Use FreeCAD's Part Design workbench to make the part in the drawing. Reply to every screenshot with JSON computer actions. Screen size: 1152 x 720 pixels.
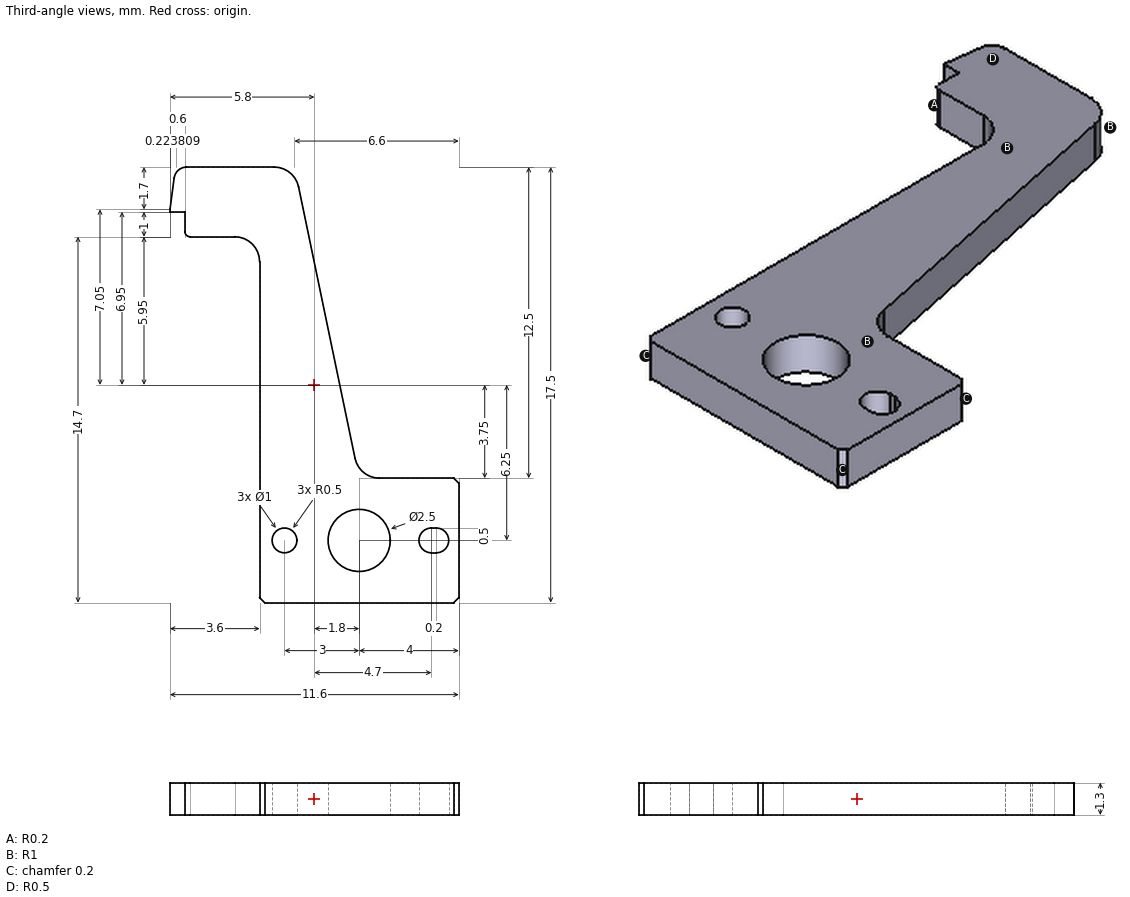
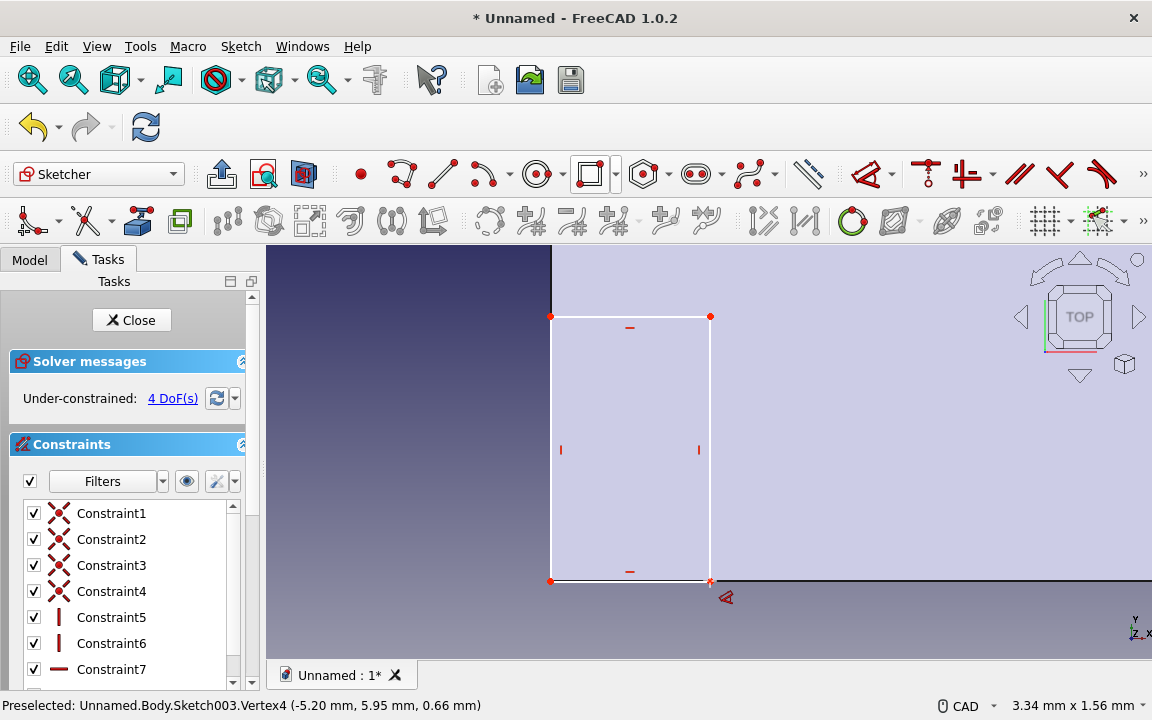
{"action": "left_click", "coordinate": [551, 396]}
{"action": "left_click", "coordinate": [517, 449]}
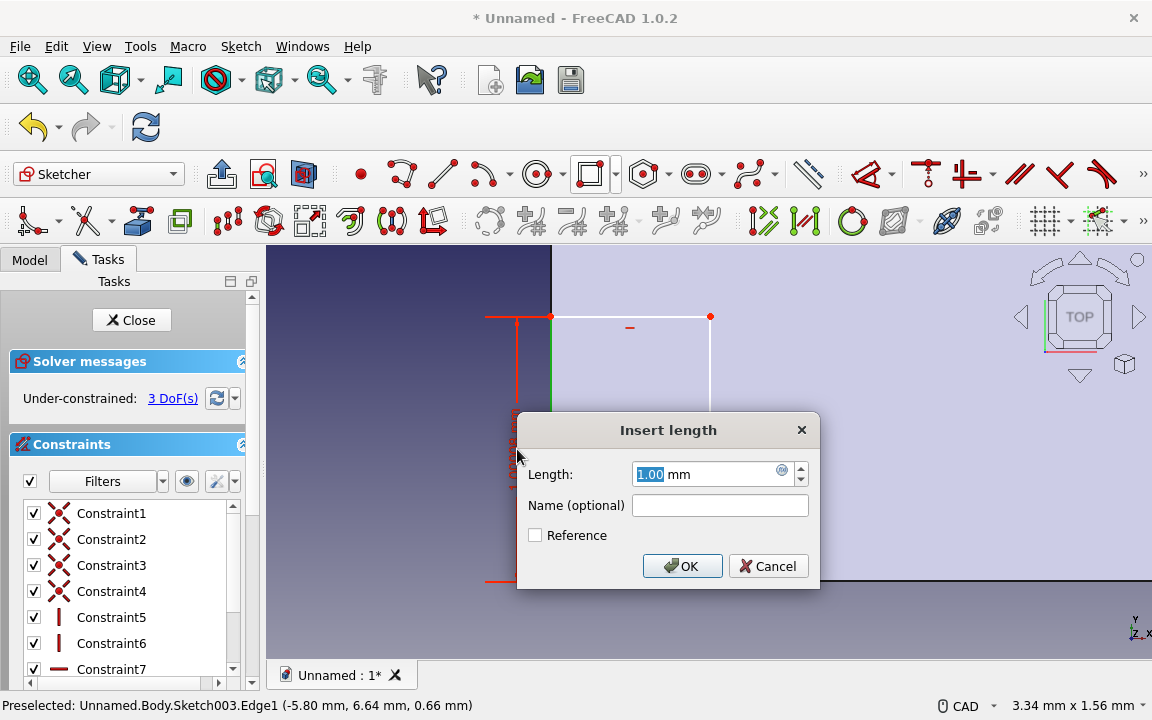
{"action": "type", "text": "1"}
{"action": "key", "text": "Return"}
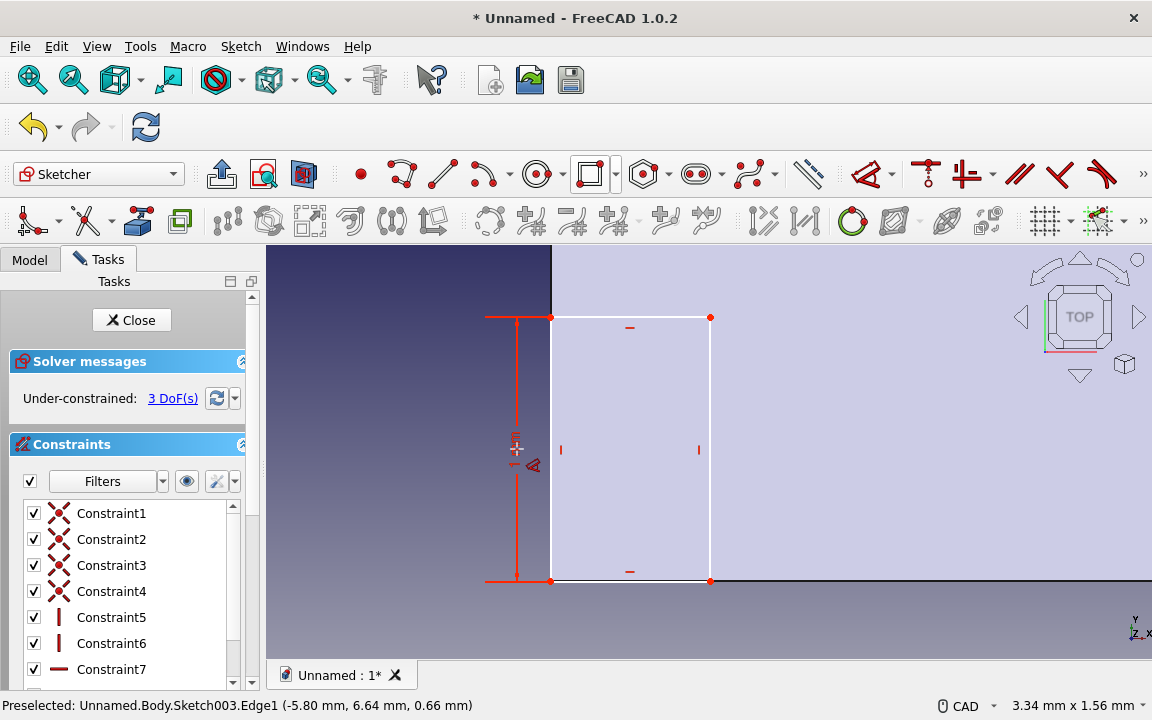
{"action": "left_click", "coordinate": [599, 582]}
{"action": "left_click", "coordinate": [630, 616]}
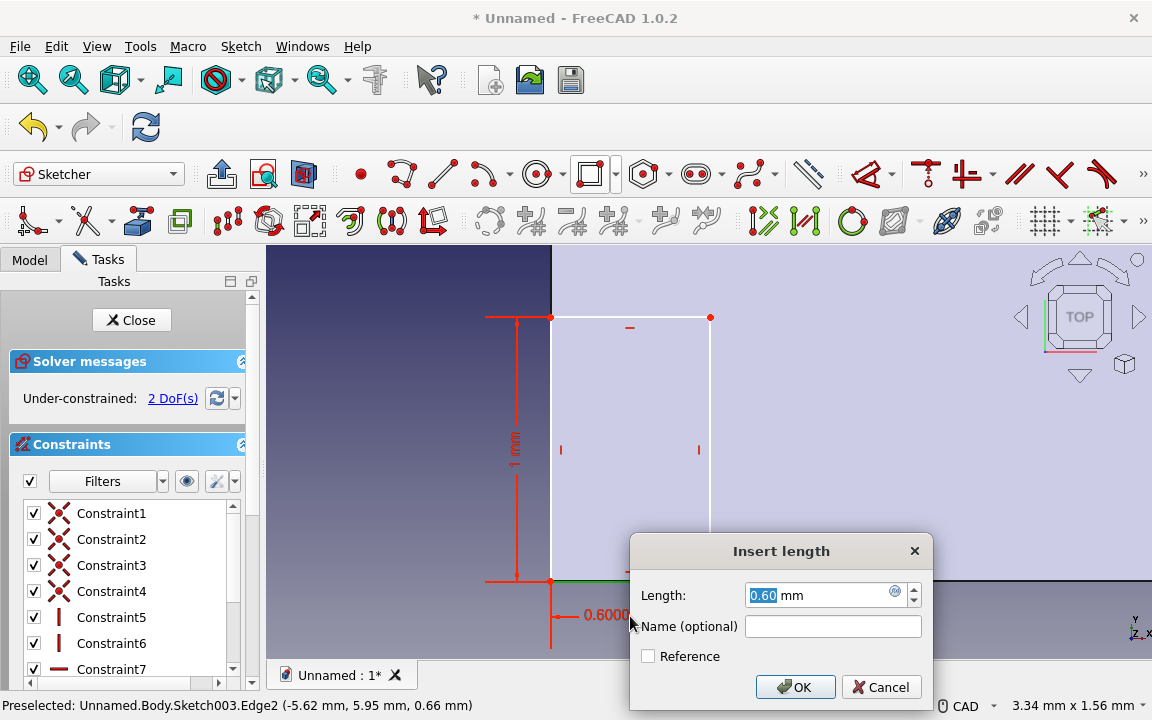
{"action": "type", "text": "0.6"}
{"action": "key", "text": "Return"}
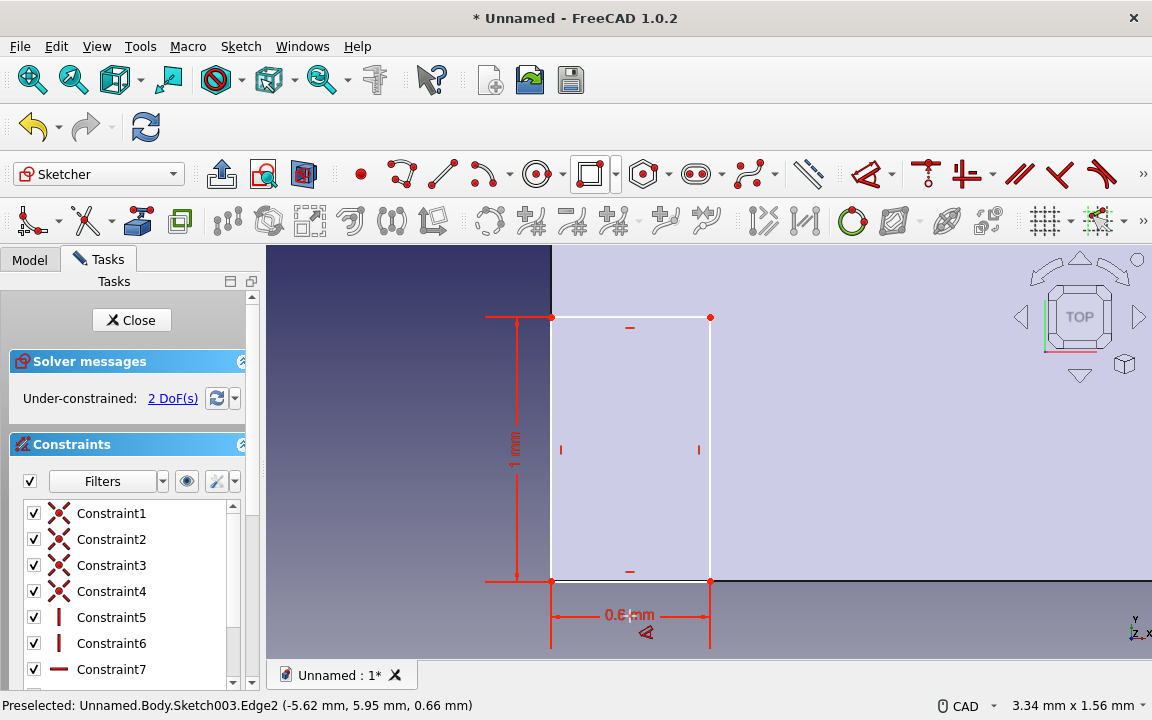
{"action": "left_click", "coordinate": [551, 317]}
{"action": "left_click", "coordinate": [769, 283]}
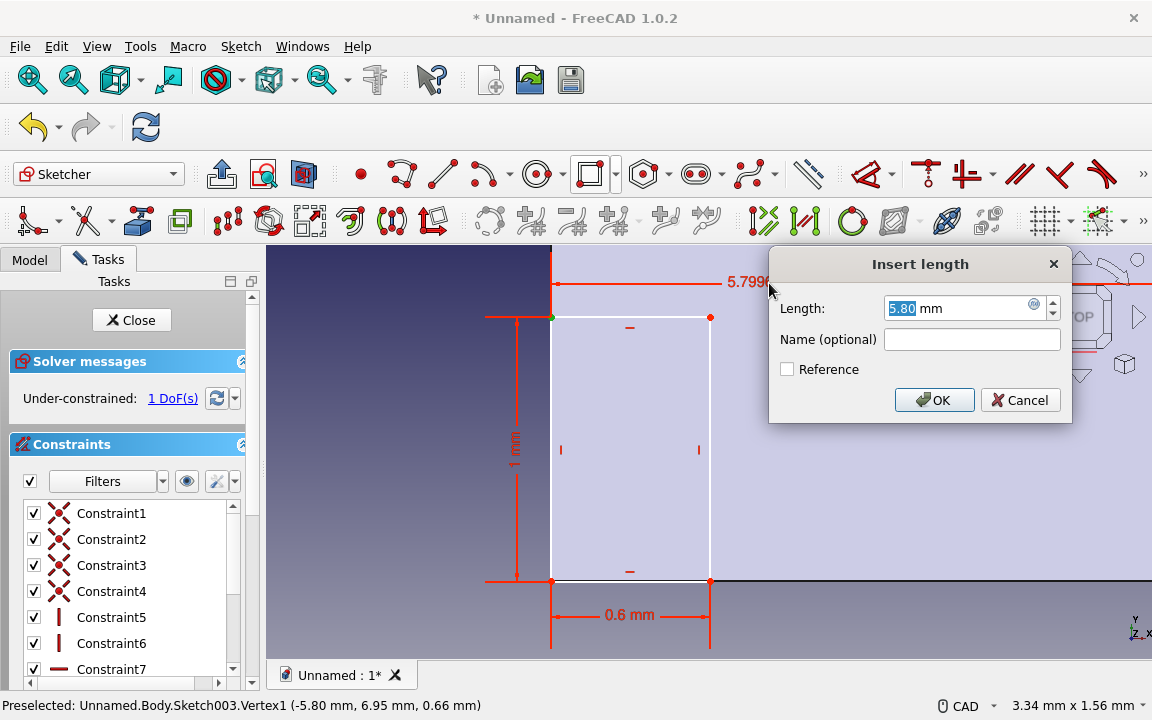
{"action": "type", "text": "5.8"}
{"action": "key", "text": "Return"}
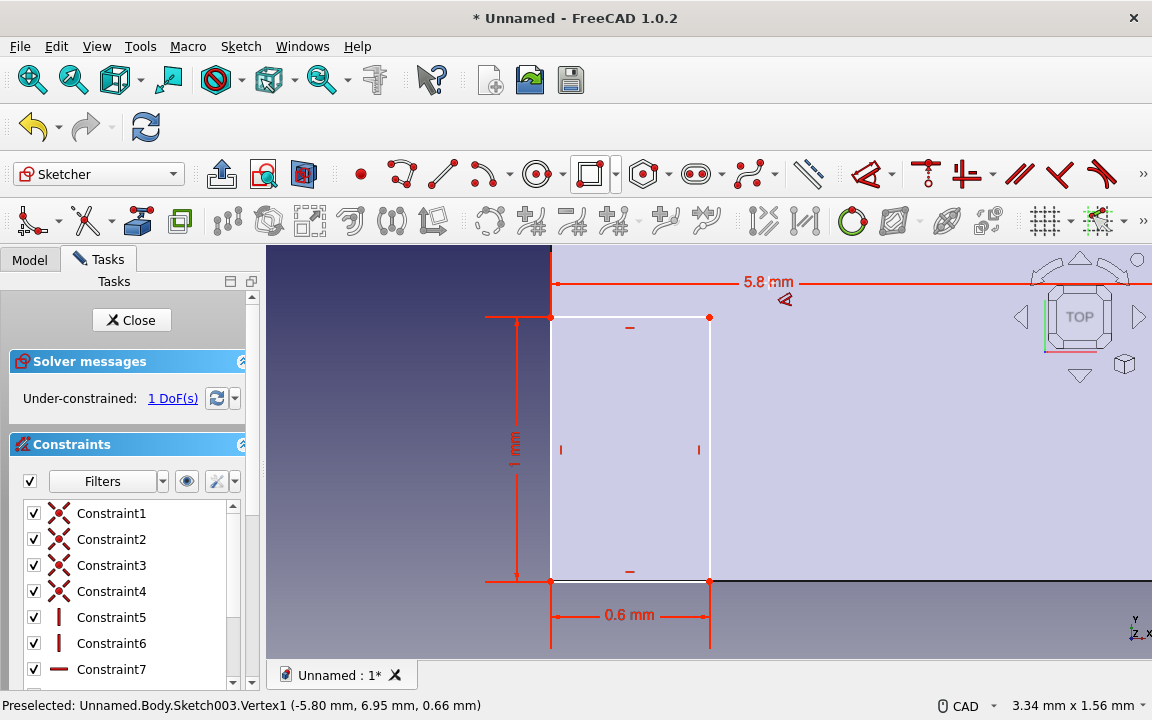
{"action": "left_click", "coordinate": [551, 317]}
{"action": "left_click", "coordinate": [517, 474]}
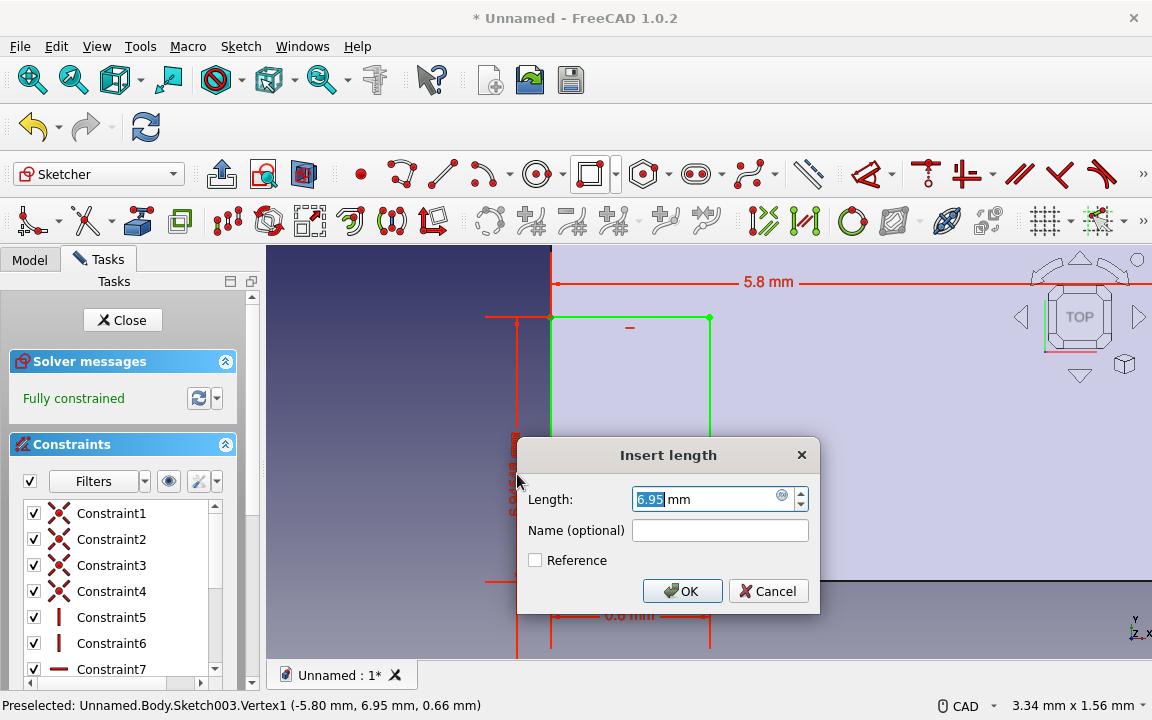
{"action": "type", "text": "6.95"}
{"action": "key", "text": "Return"}
{"action": "key", "text": "Escape"}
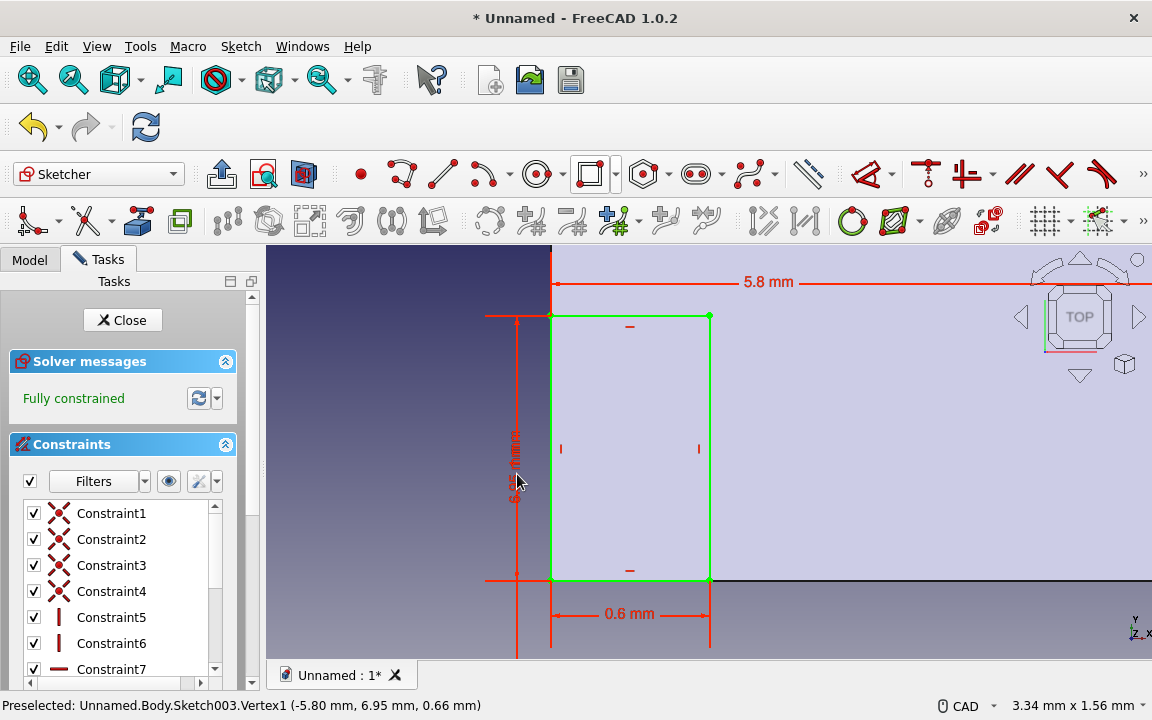
{"action": "left_click", "coordinate": [123, 320]}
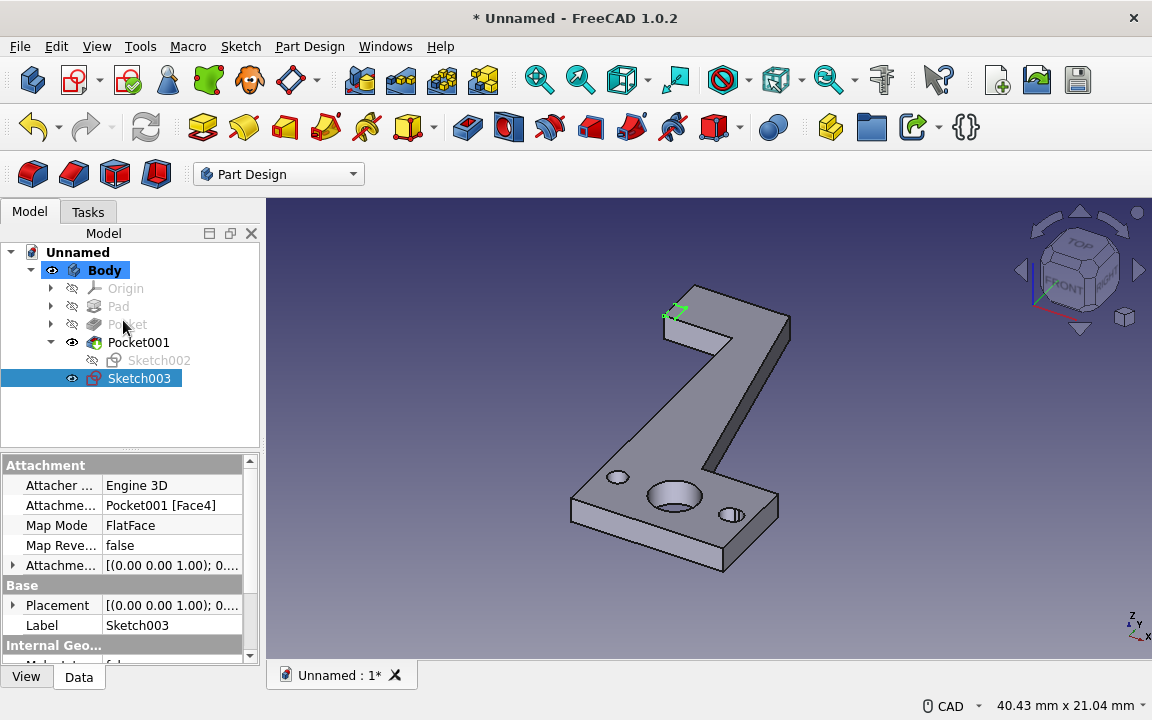
{"action": "left_click", "coordinate": [468, 128]}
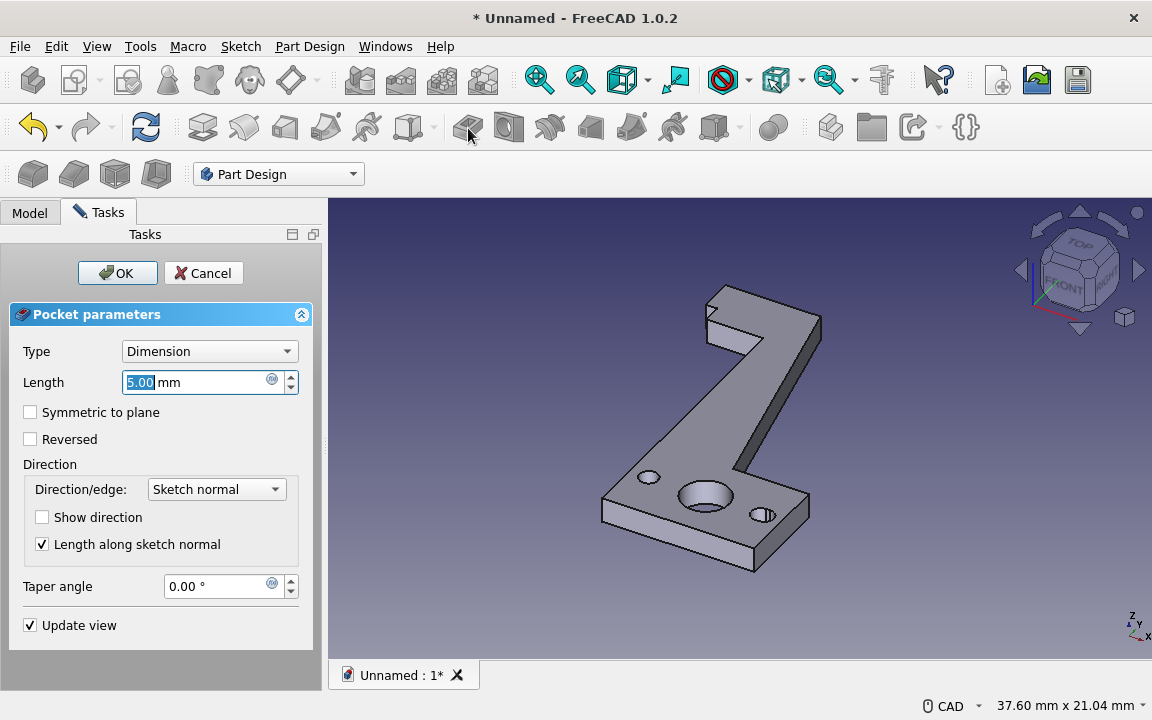
{"action": "left_click", "coordinate": [210, 352]}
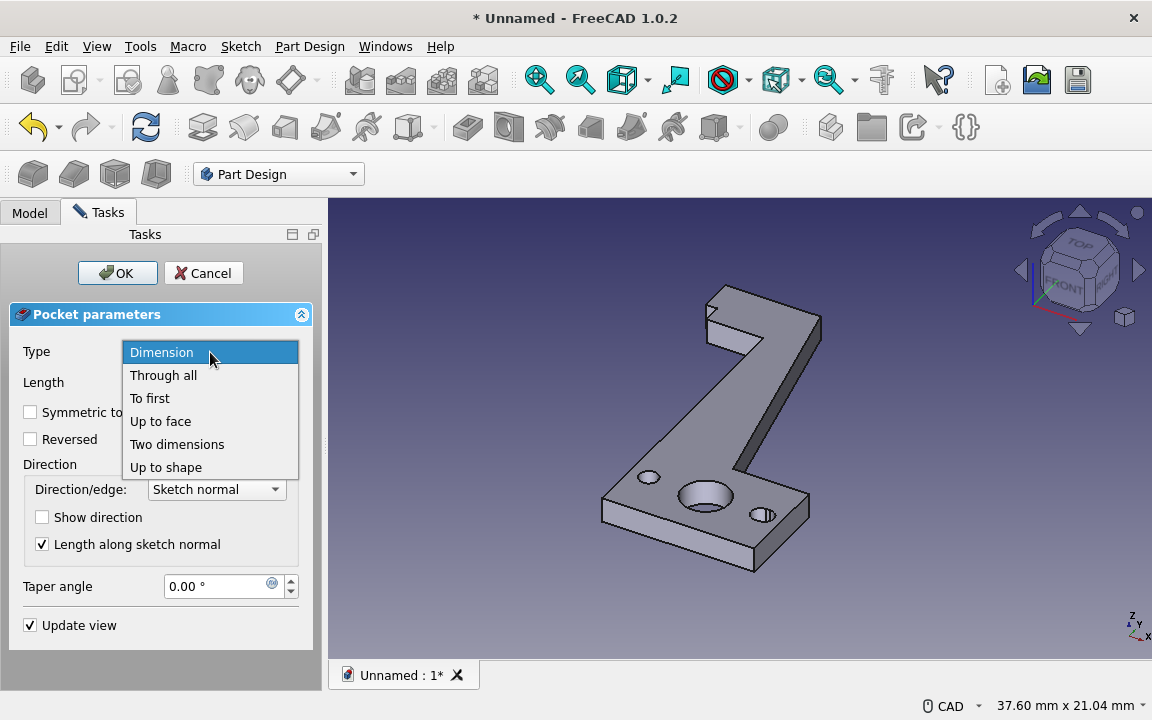
{"action": "left_click", "coordinate": [208, 376]}